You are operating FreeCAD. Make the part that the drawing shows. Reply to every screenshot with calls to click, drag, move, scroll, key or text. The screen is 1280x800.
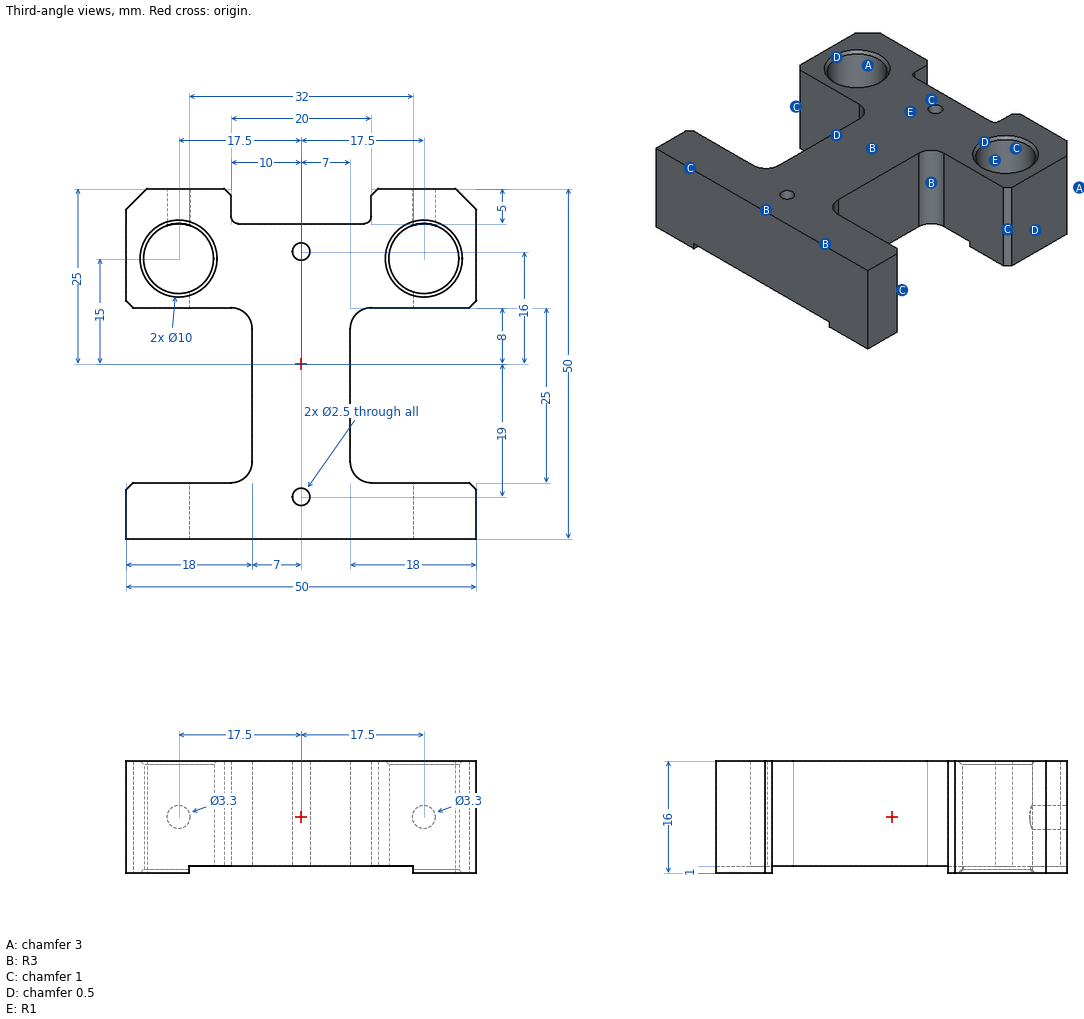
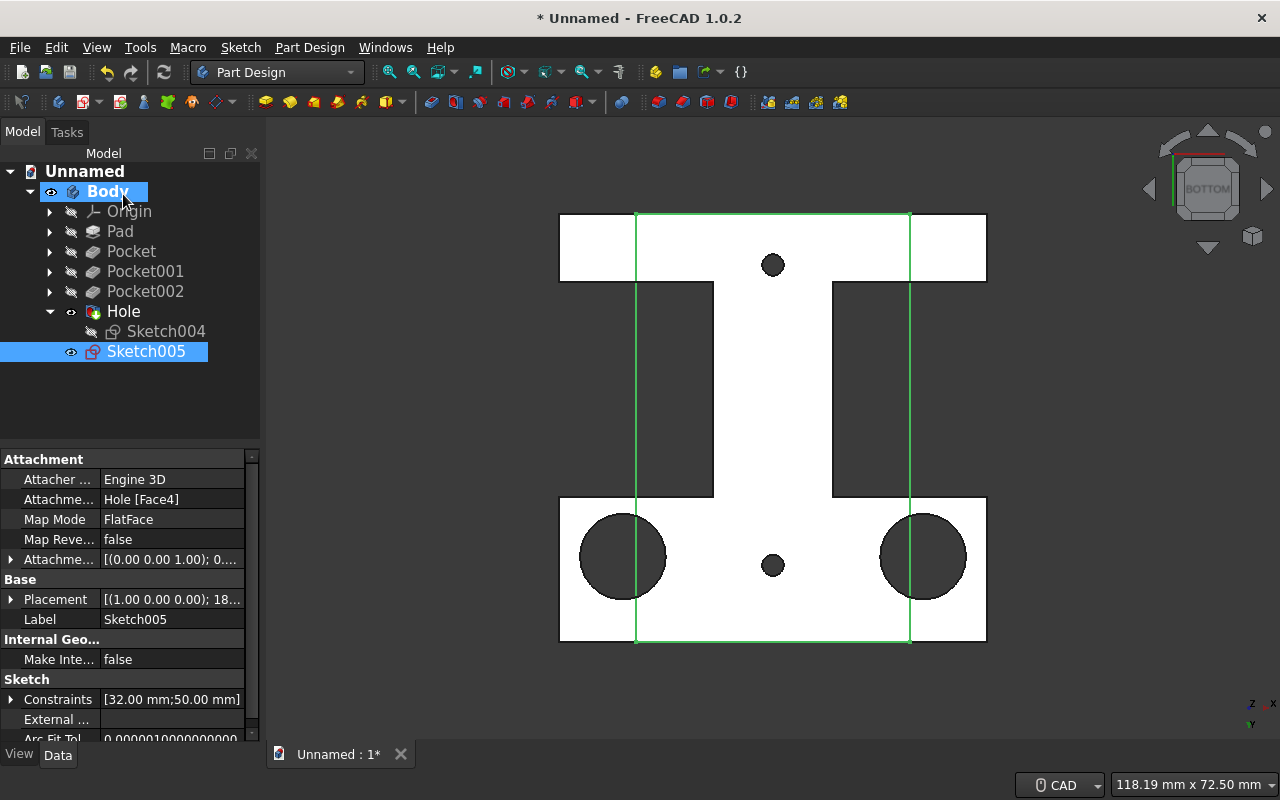
click(432, 102)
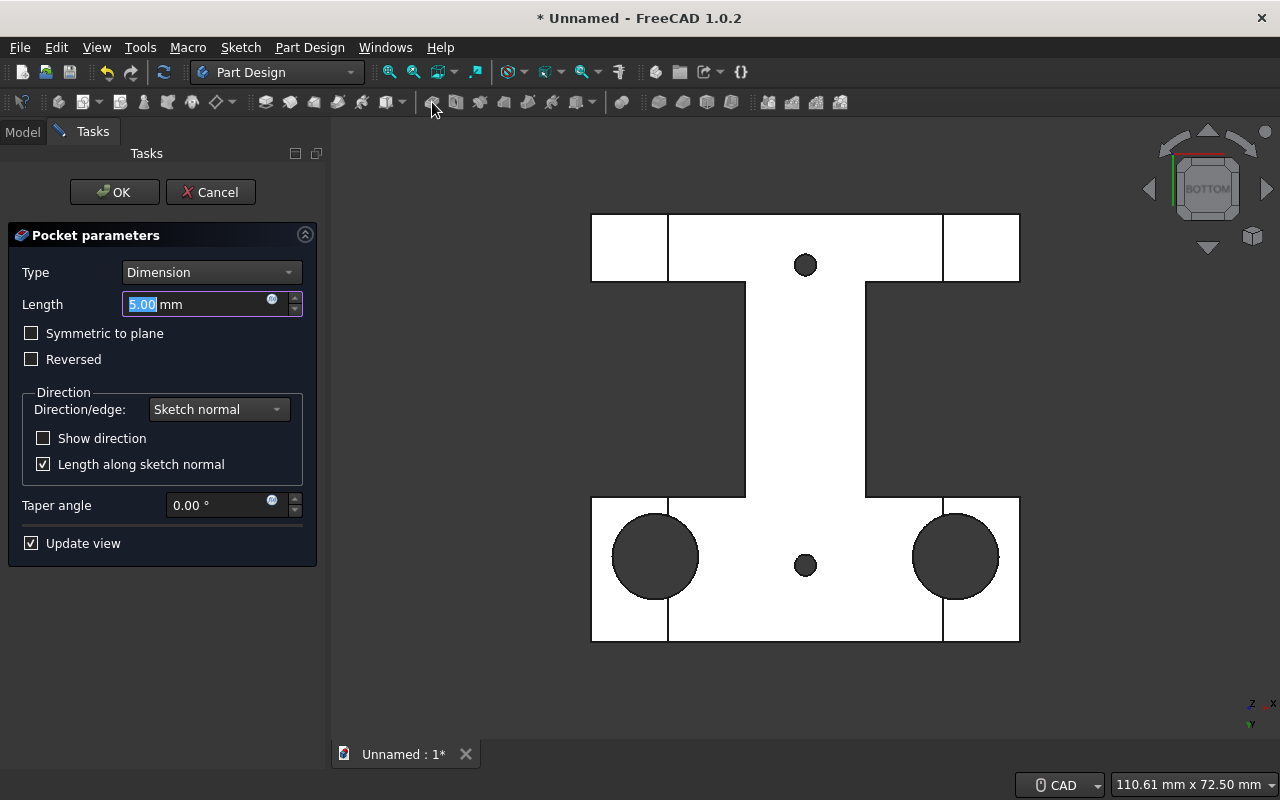
text(1)
key(Tab)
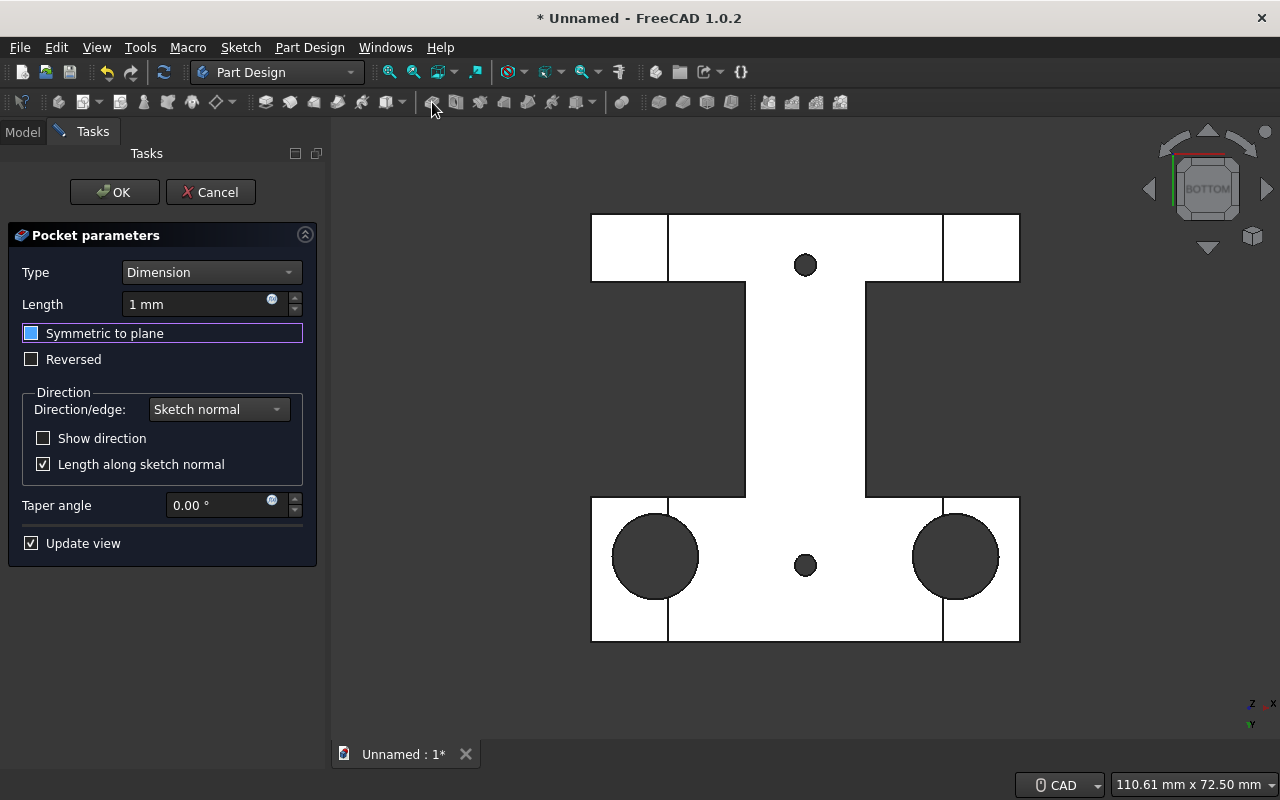
click(115, 192)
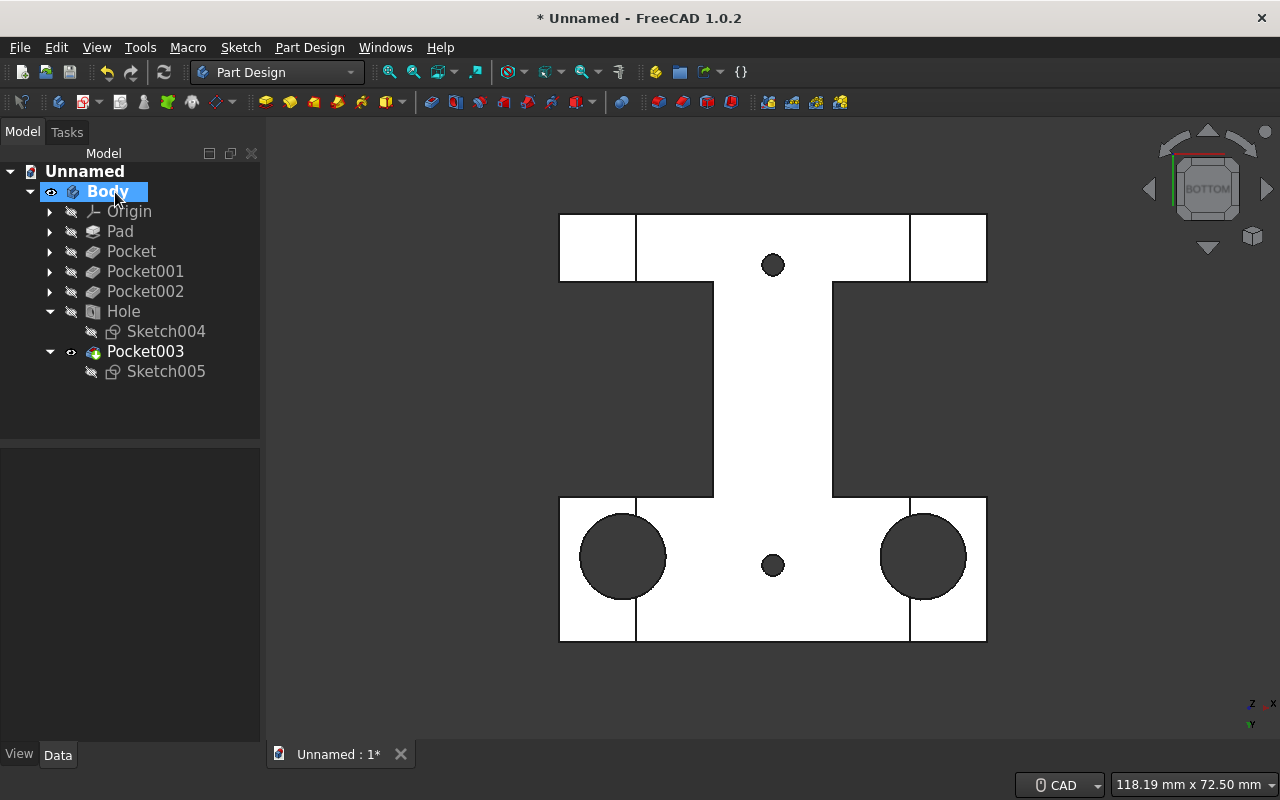
key(0)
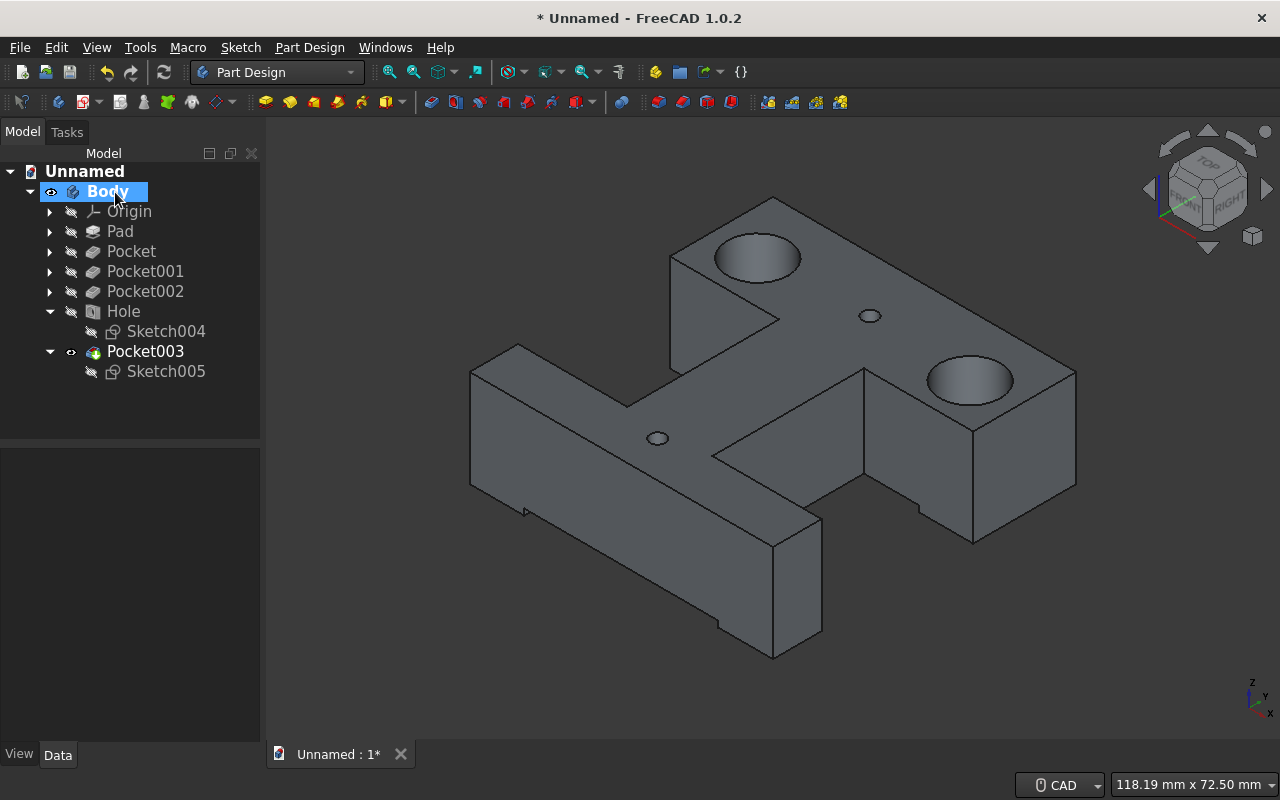
click(816, 346)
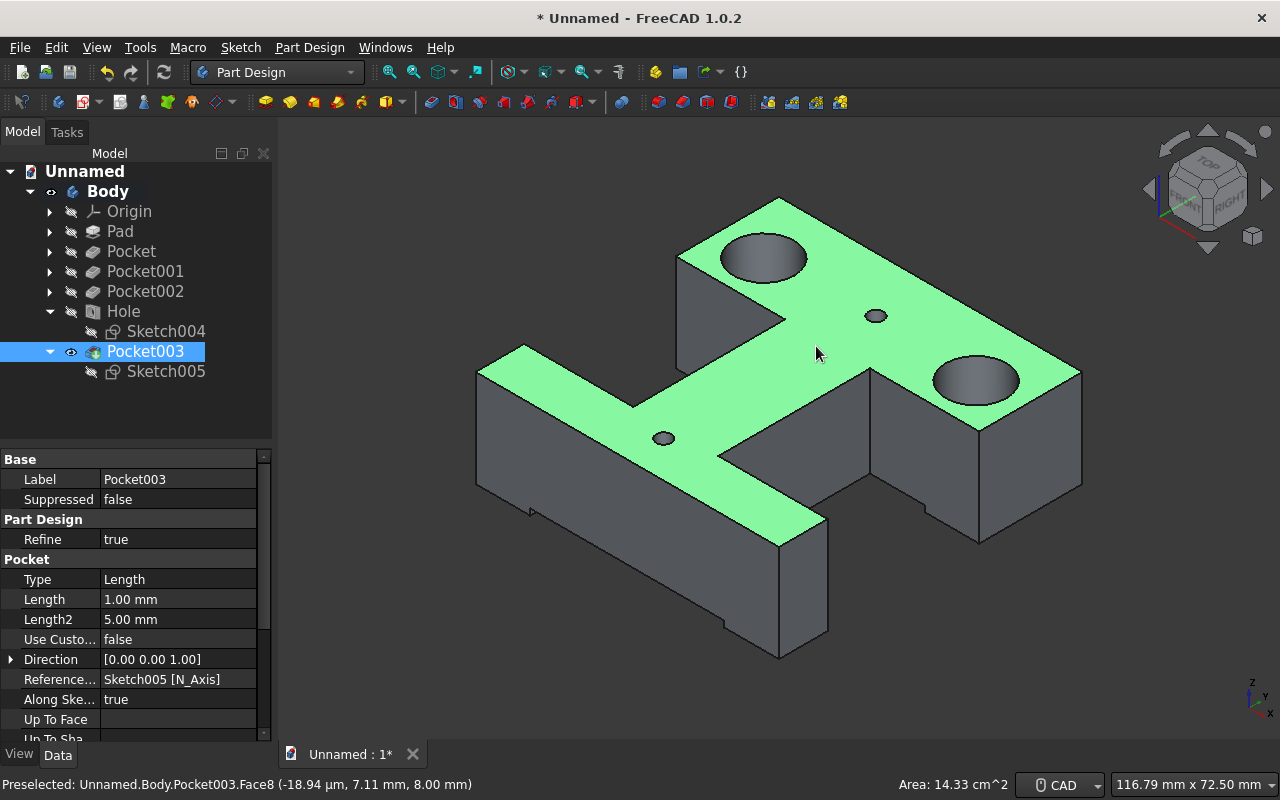
click(84, 102)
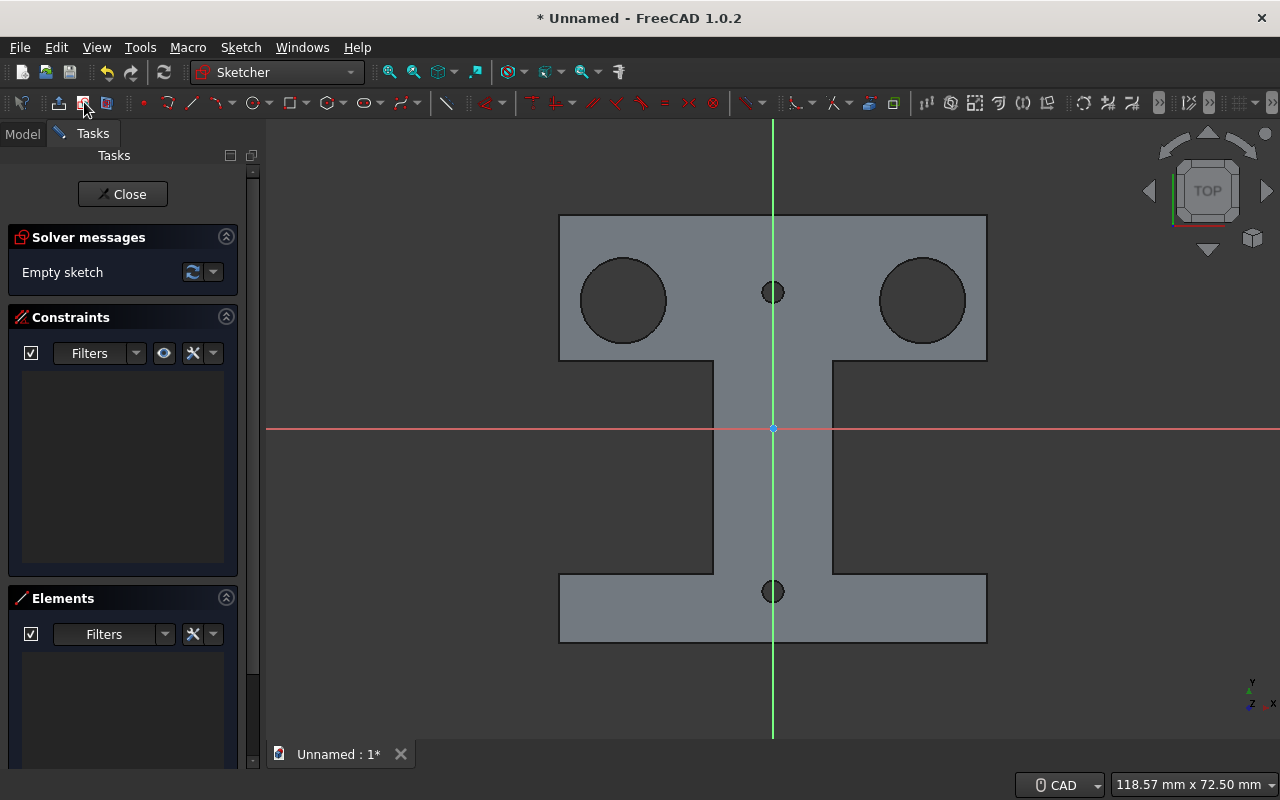
scroll(856, 192, up, 3)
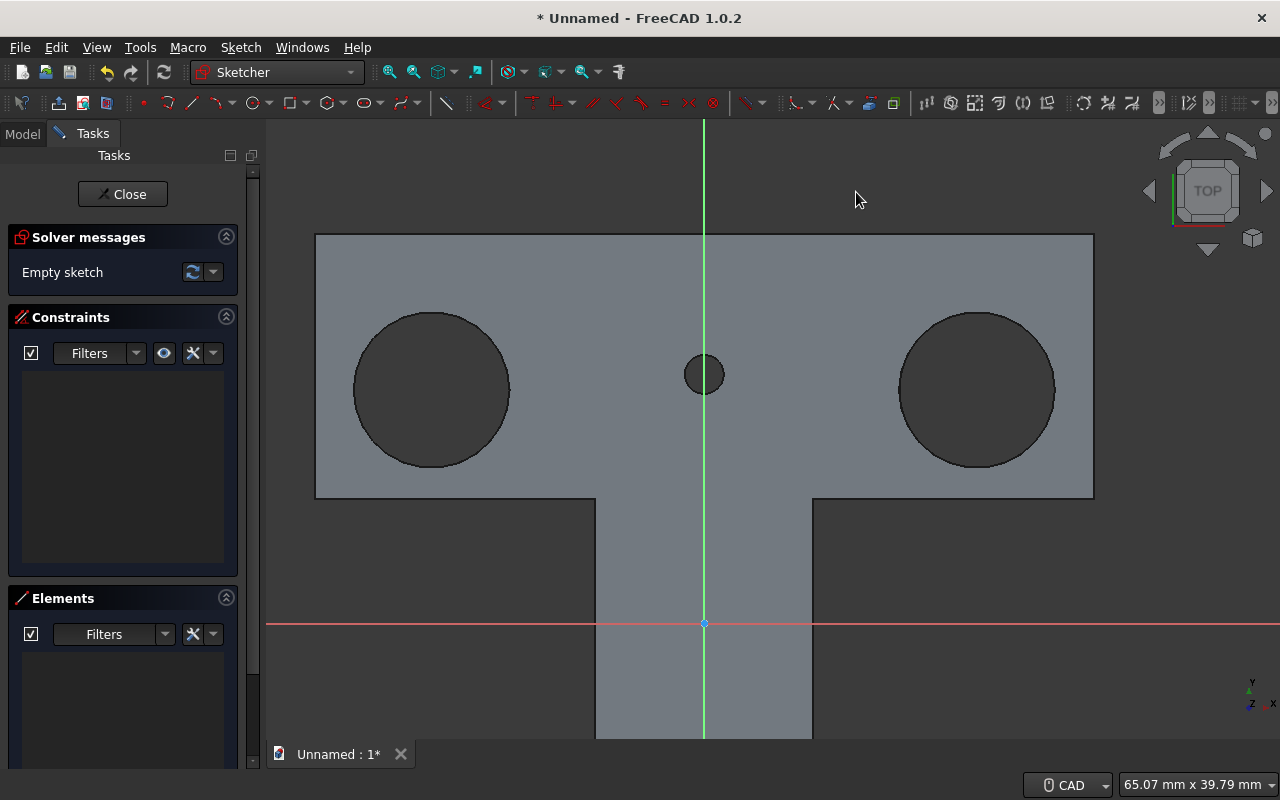
key(g)
key(r)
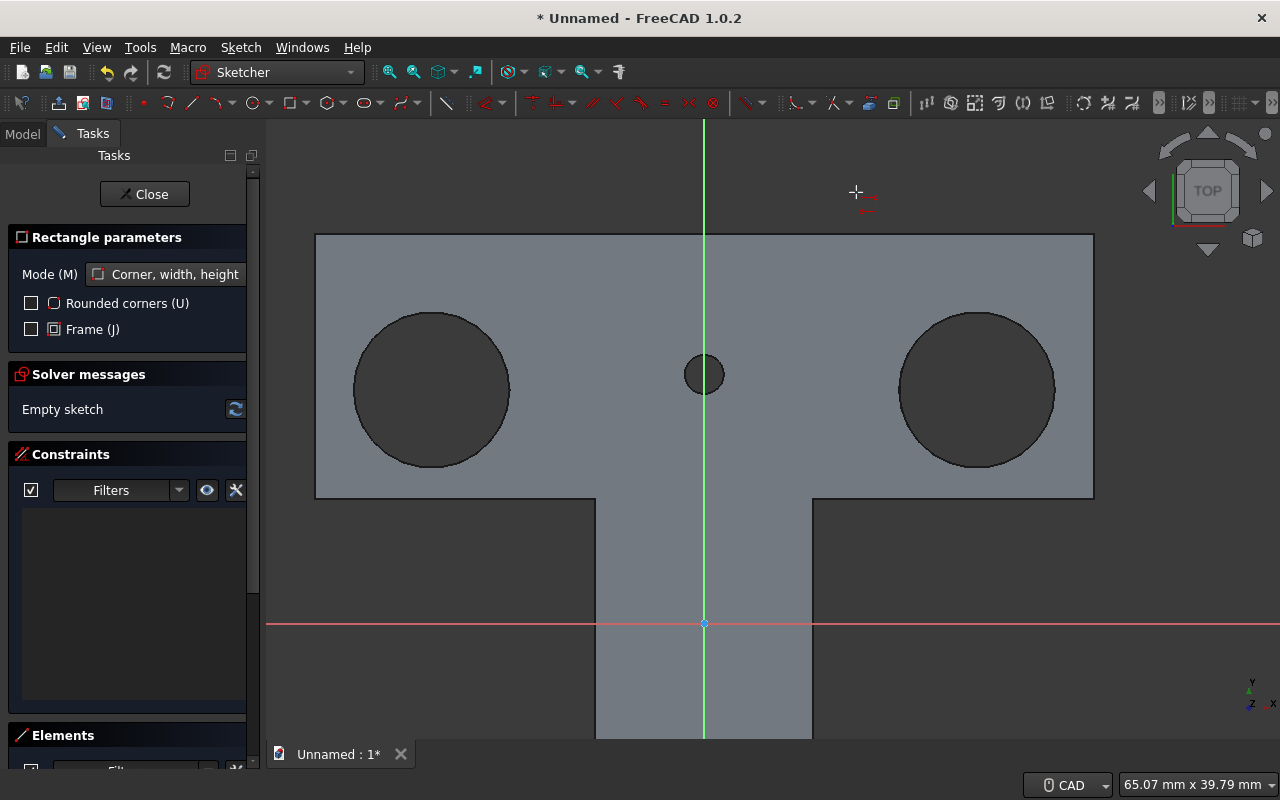
click(548, 234)
move(860, 312)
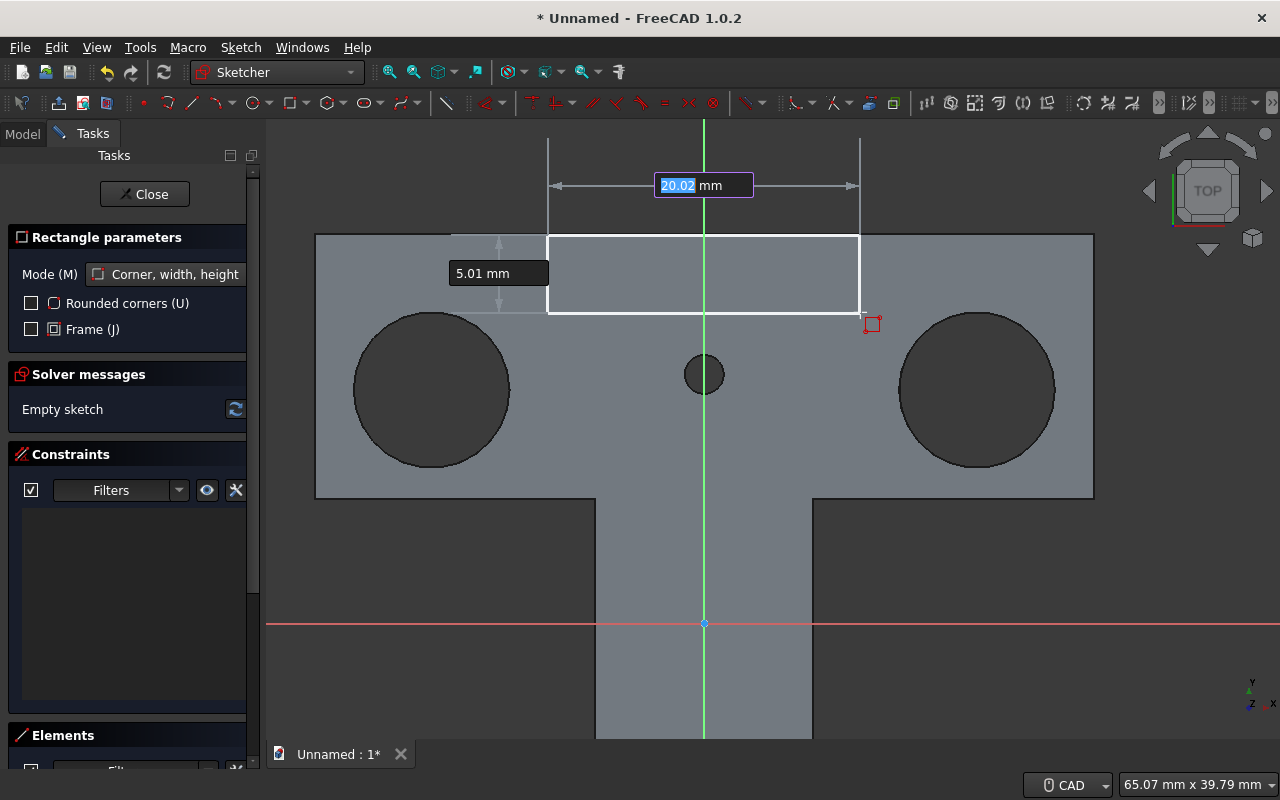
text(20)
key(Tab)
text(5)
key(Return)
key(Escape)